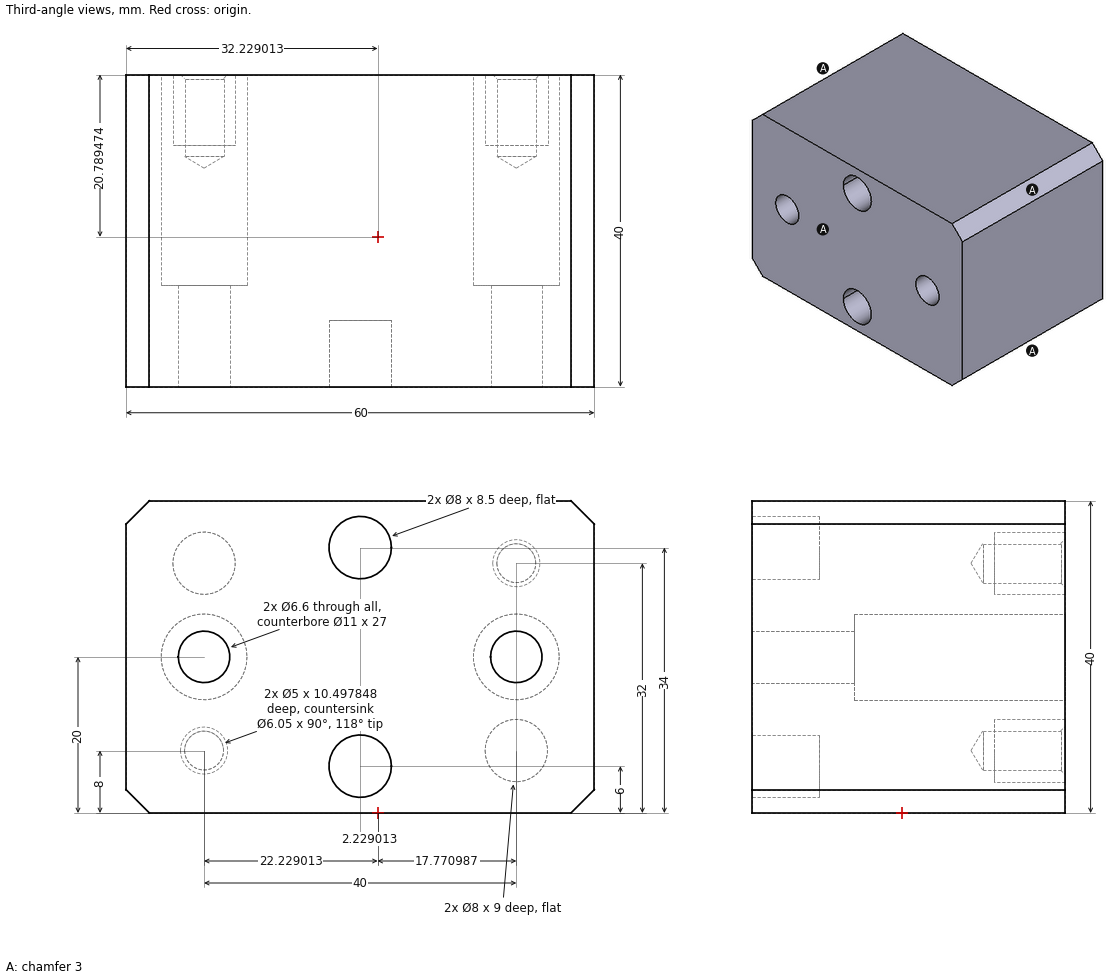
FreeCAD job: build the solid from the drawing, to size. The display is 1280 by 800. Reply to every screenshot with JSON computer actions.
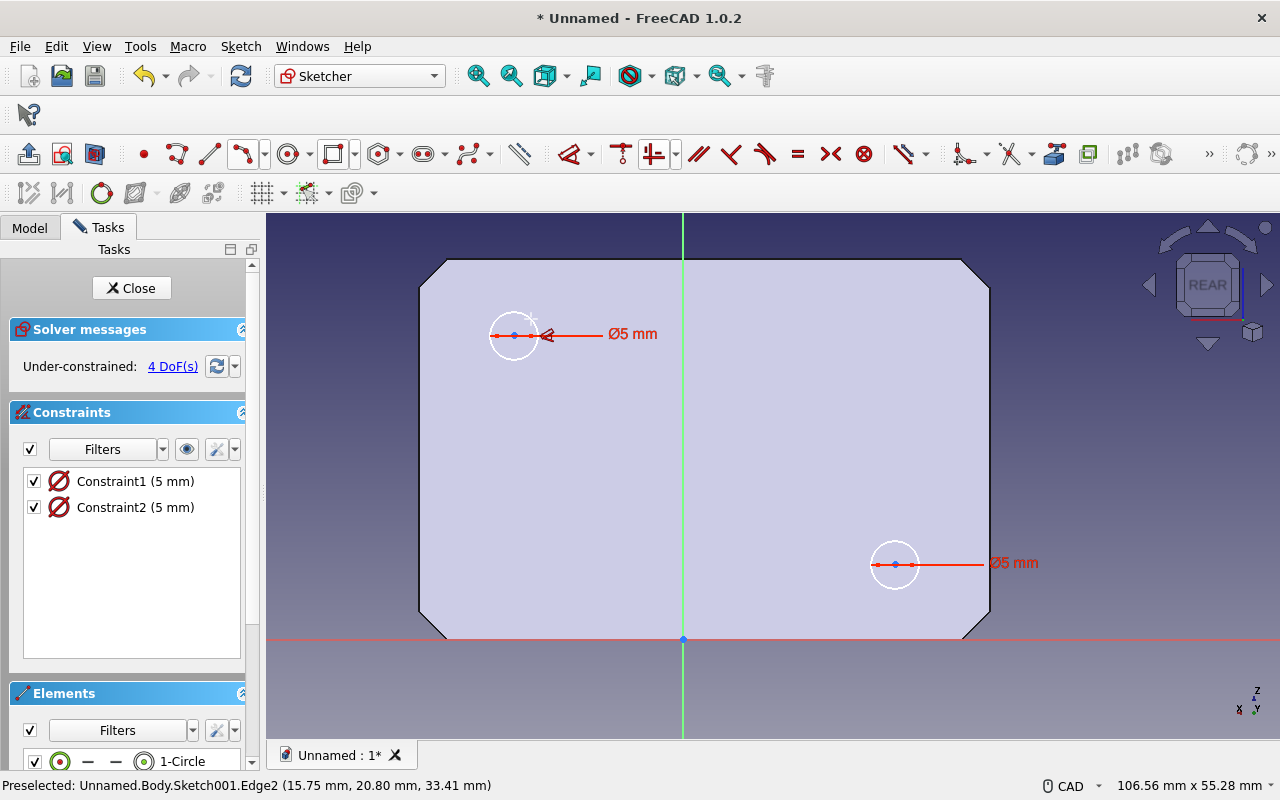
{"action": "left_click", "coordinate": [895, 565]}
{"action": "left_click", "coordinate": [929, 602]}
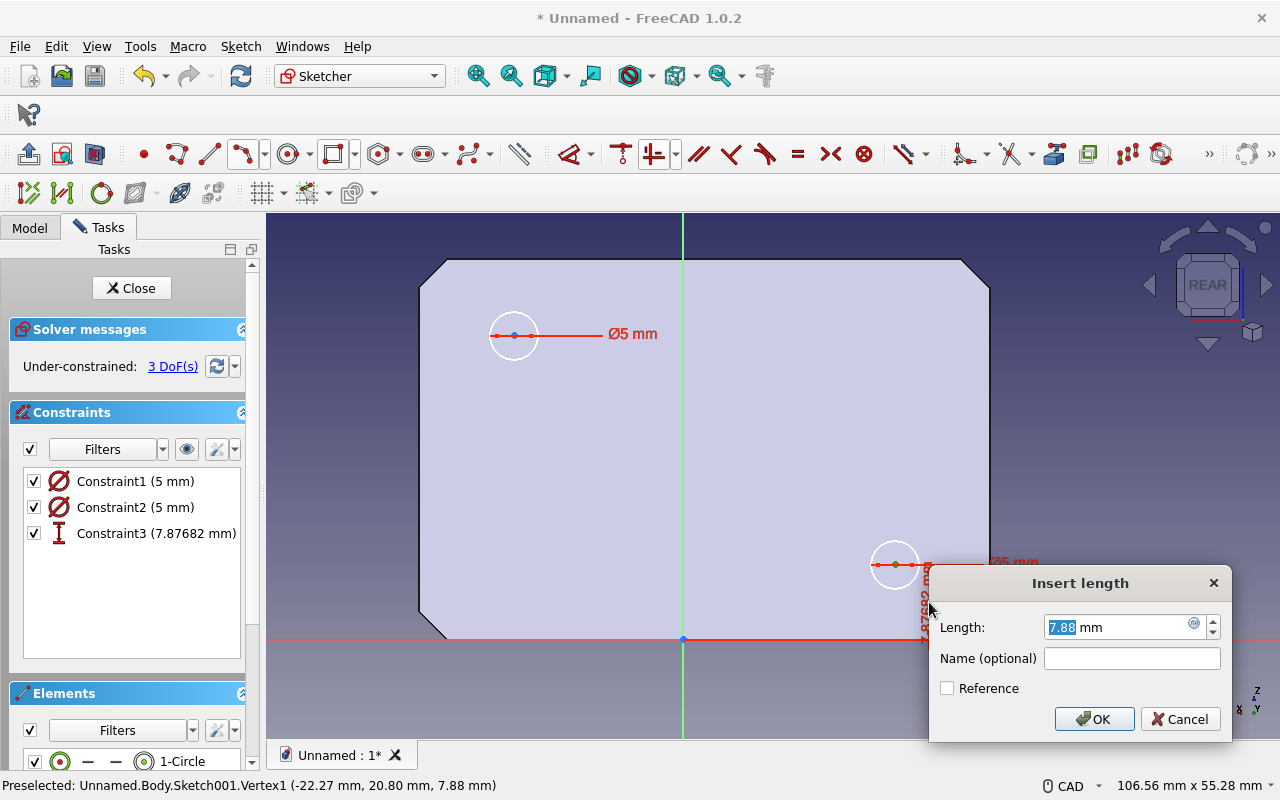
{"action": "type", "text": "8"}
{"action": "key", "text": "Return"}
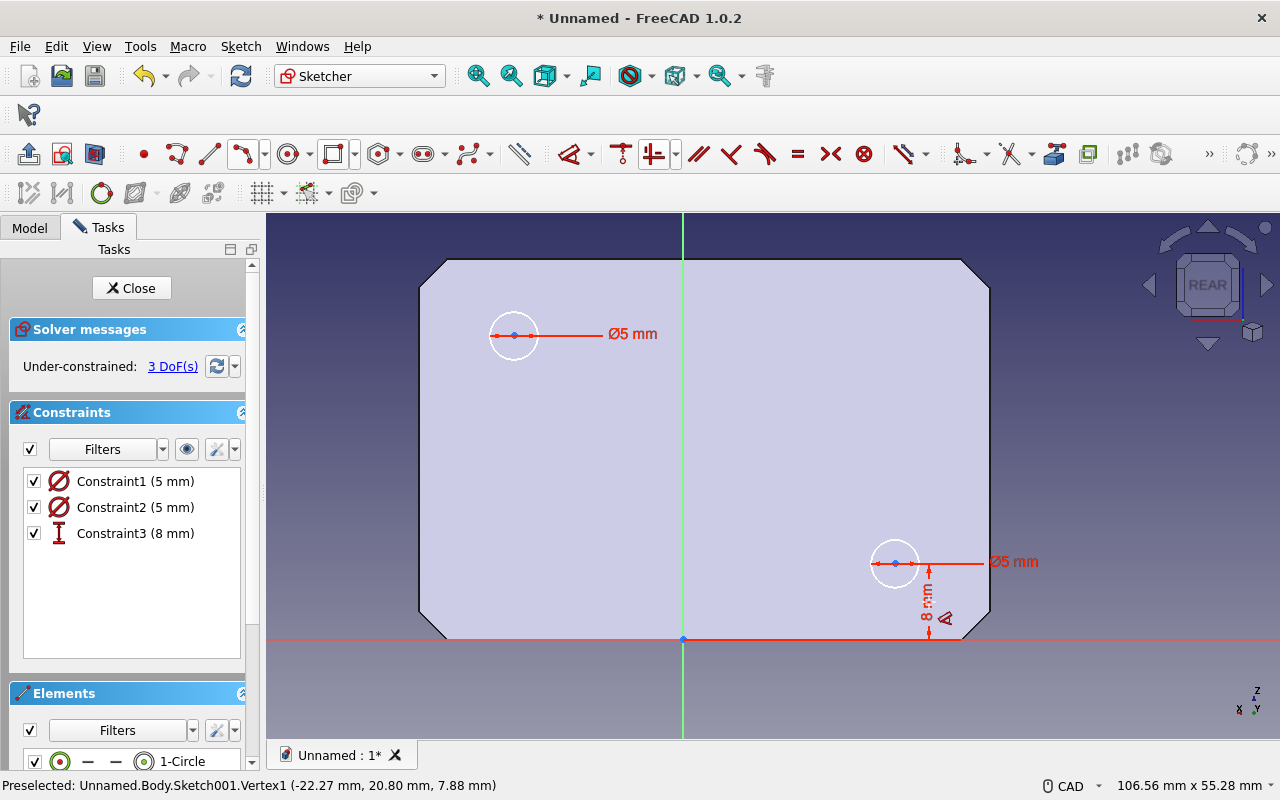
{"action": "left_click", "coordinate": [514, 336]}
{"action": "left_click", "coordinate": [480, 488]}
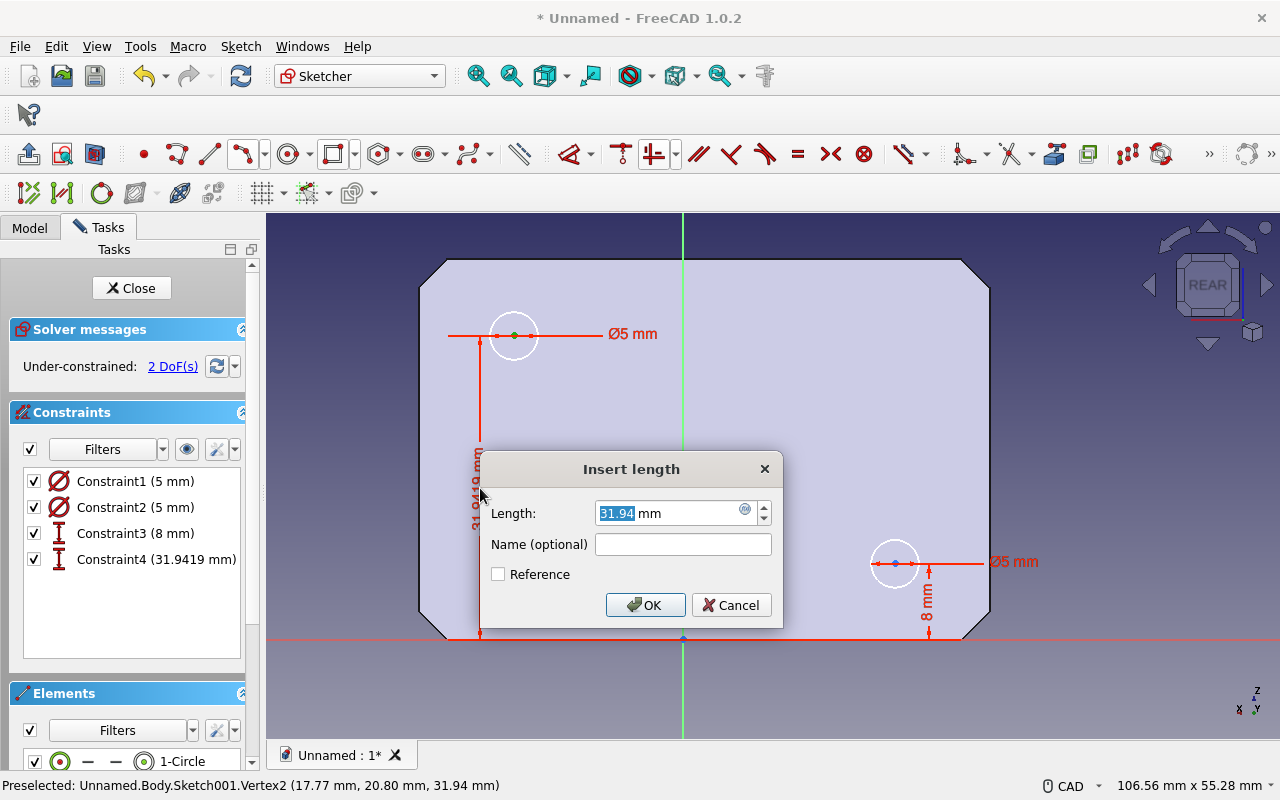
{"action": "type", "text": "32"}
{"action": "key", "text": "Return"}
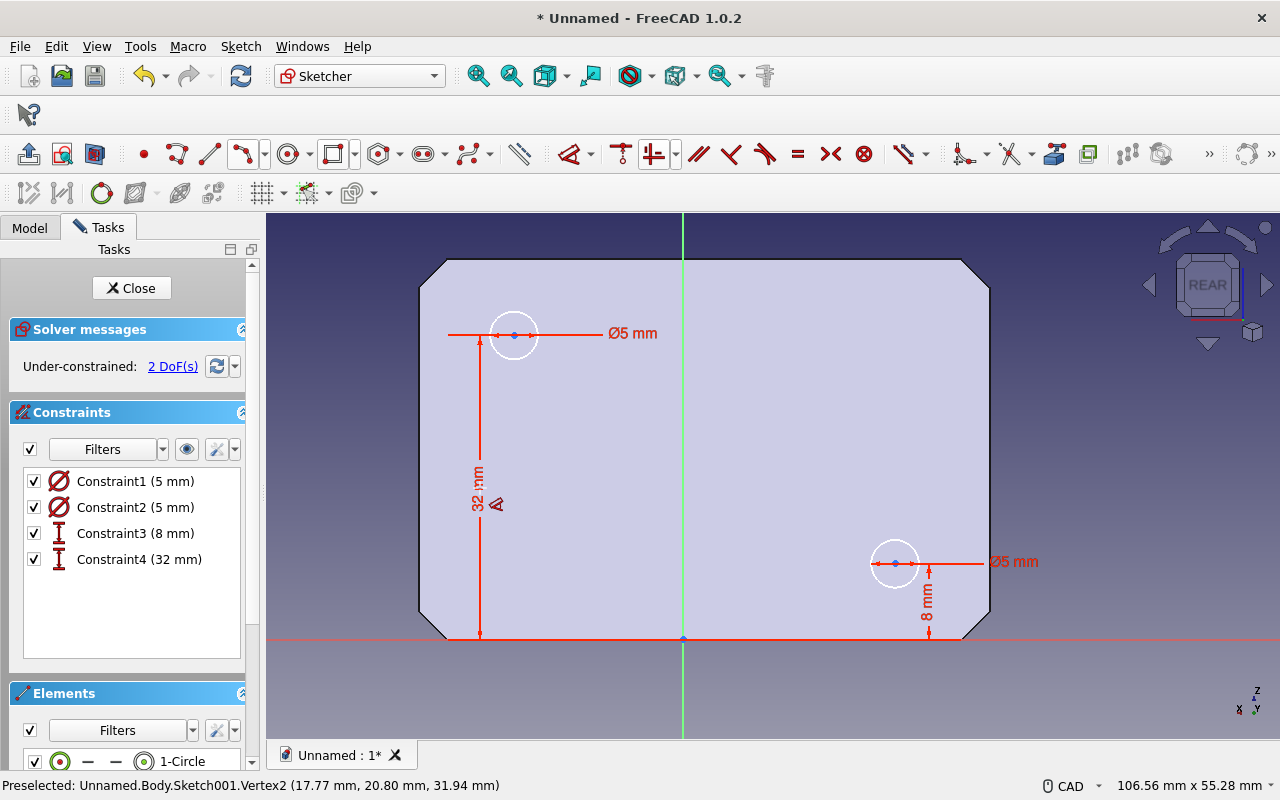
{"action": "left_click", "coordinate": [895, 564]}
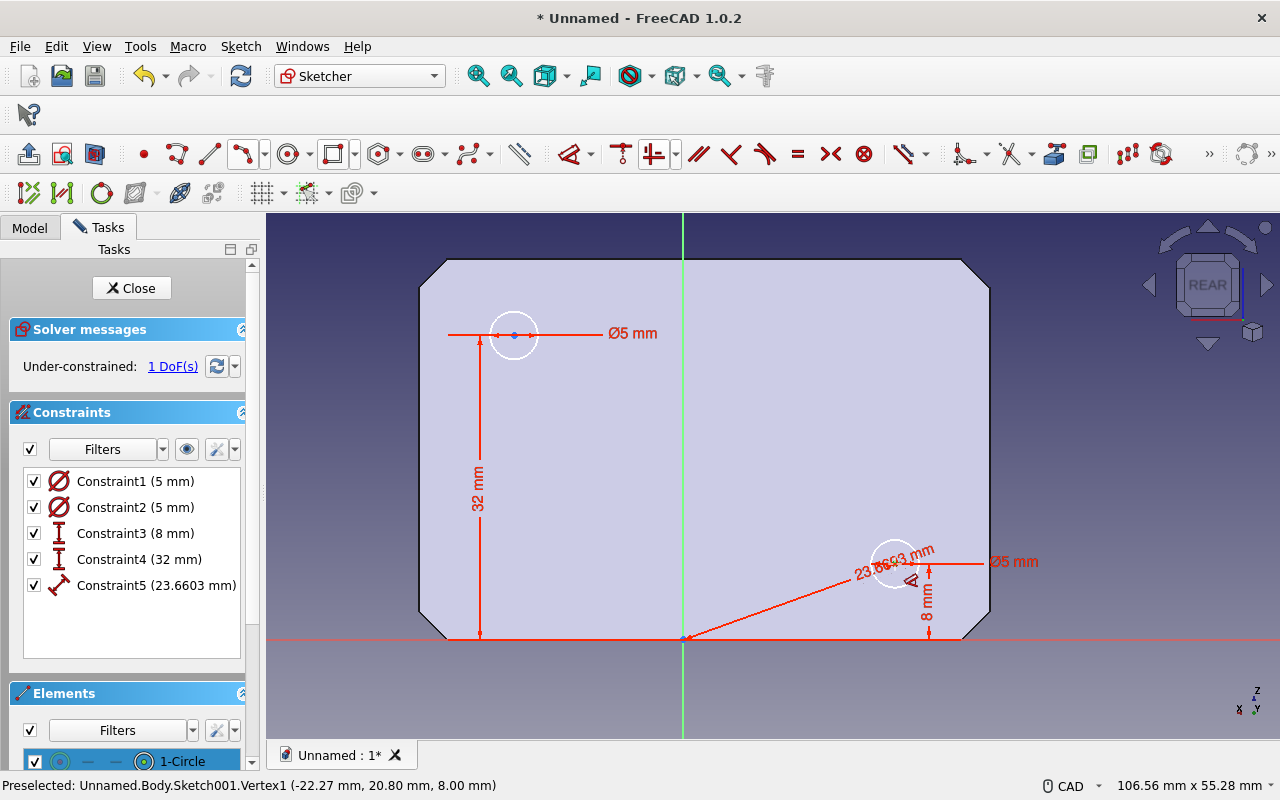
{"action": "left_click", "coordinate": [514, 335]}
{"action": "left_click", "coordinate": [704, 301]}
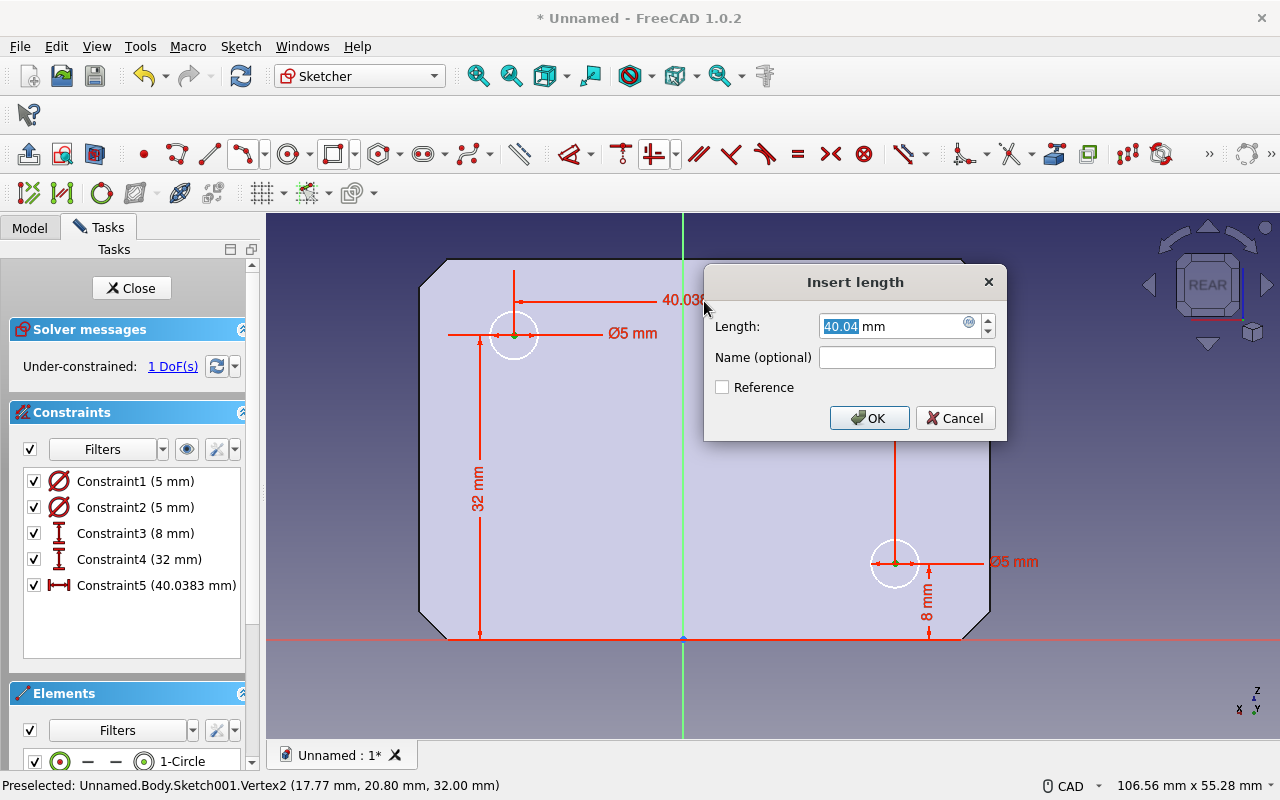
{"action": "type", "text": "40"}
{"action": "key", "text": "Return"}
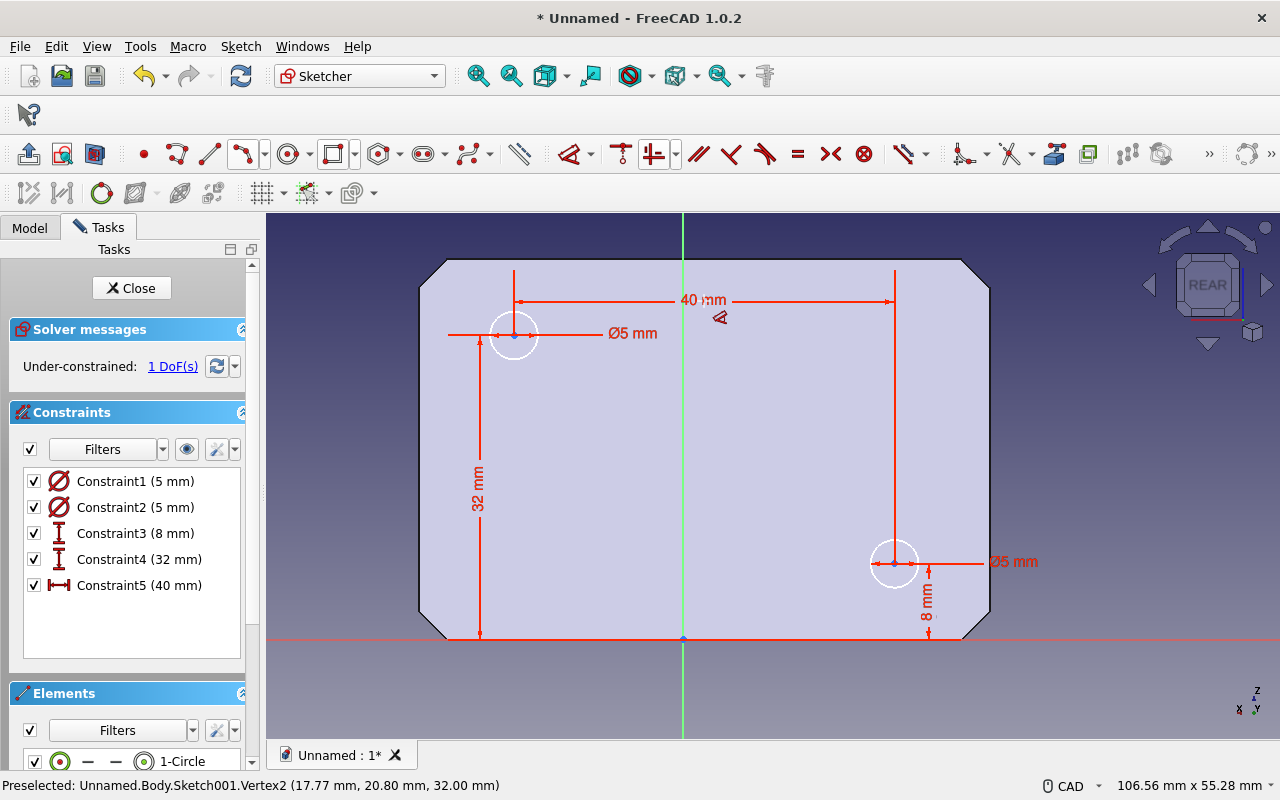
{"action": "left_click", "coordinate": [895, 564]}
{"action": "left_click", "coordinate": [789, 674]}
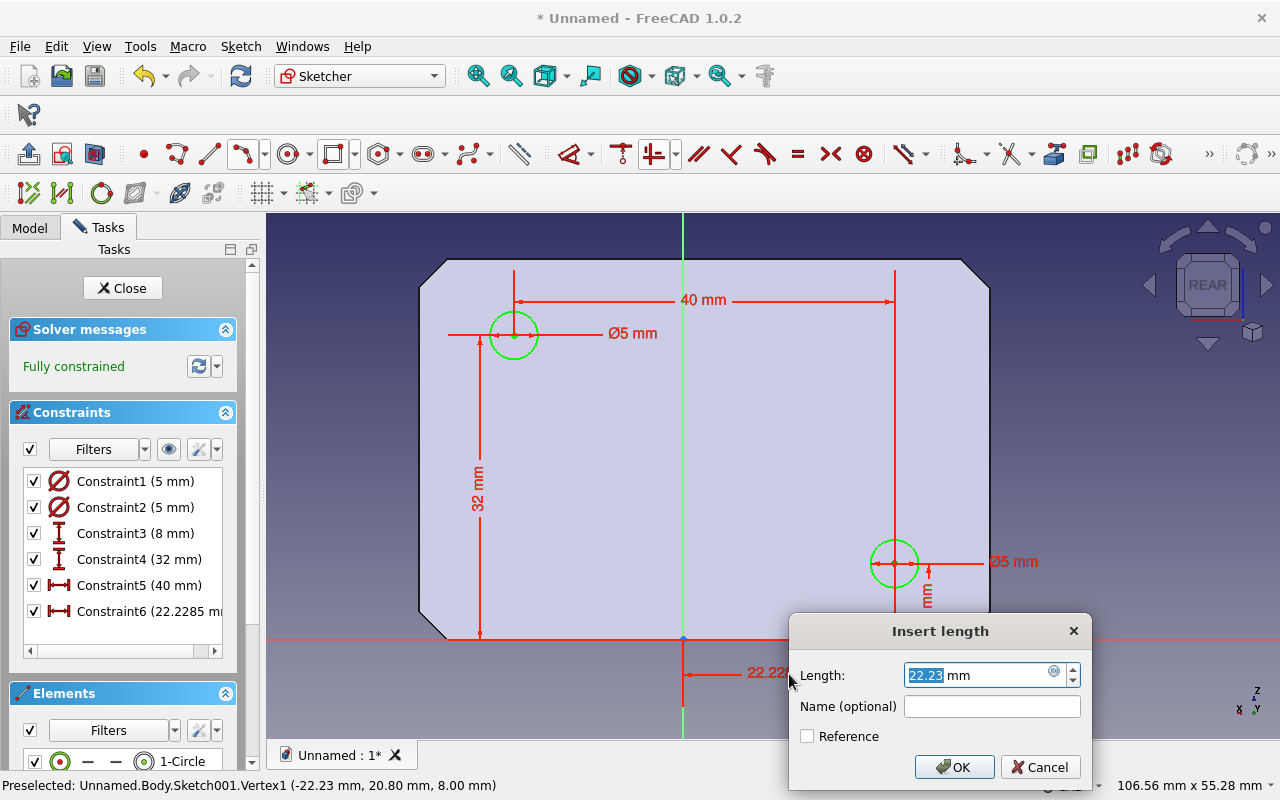
{"action": "type", "text": "22.229013"}
{"action": "key", "text": "Return"}
{"action": "key", "text": "Escape"}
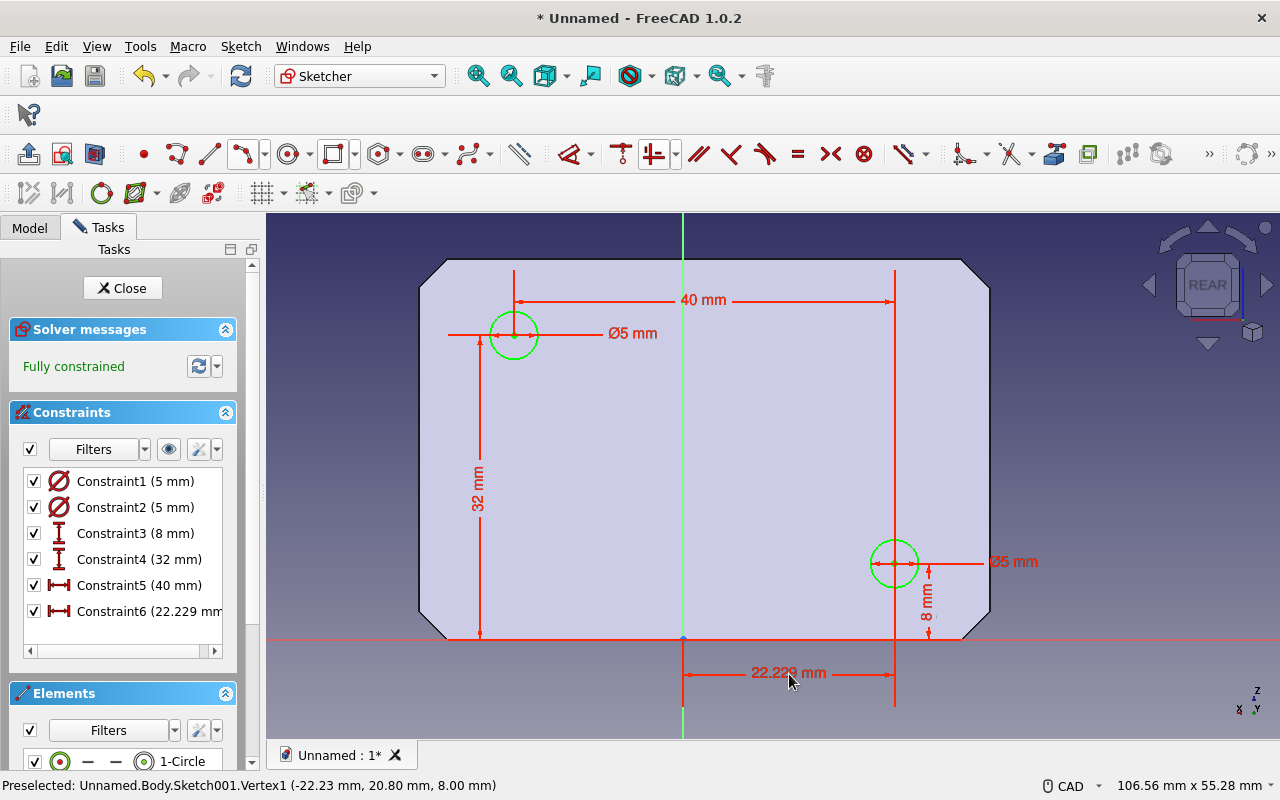
{"action": "left_click", "coordinate": [123, 288]}